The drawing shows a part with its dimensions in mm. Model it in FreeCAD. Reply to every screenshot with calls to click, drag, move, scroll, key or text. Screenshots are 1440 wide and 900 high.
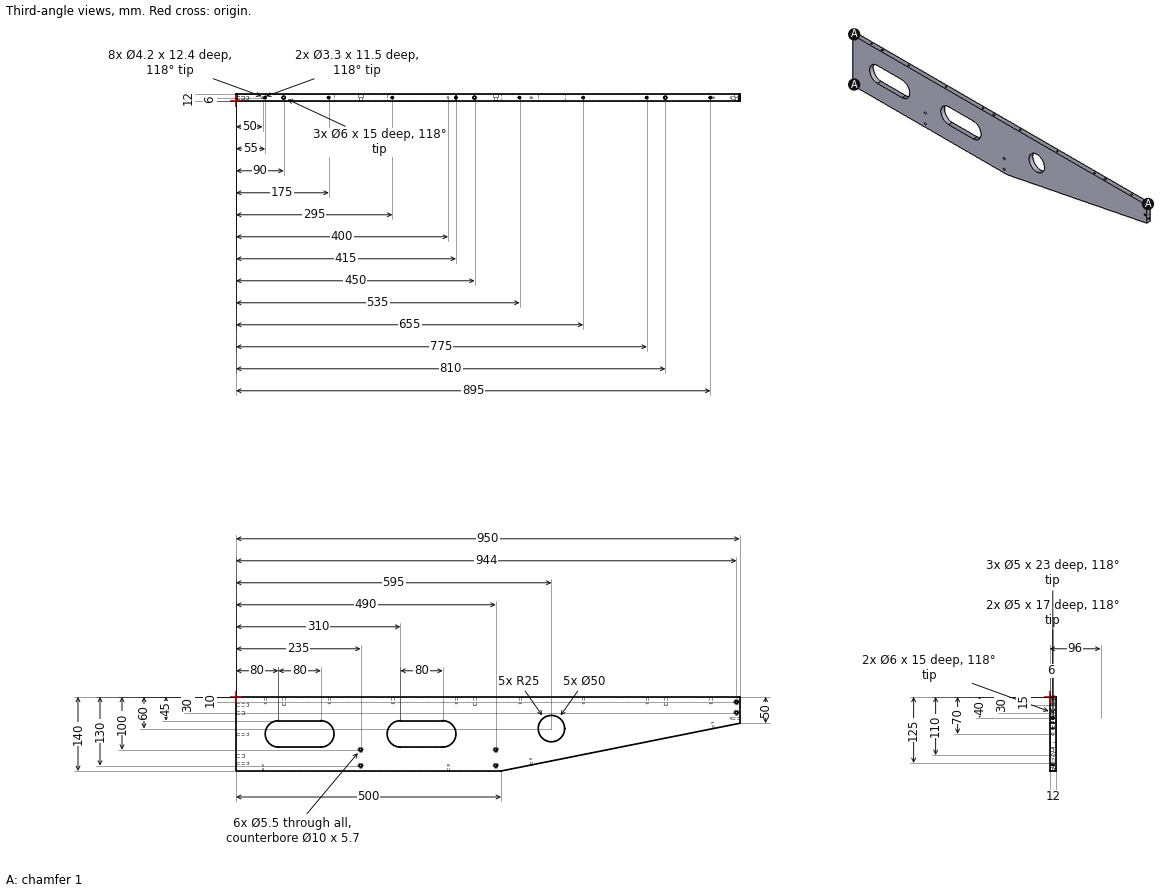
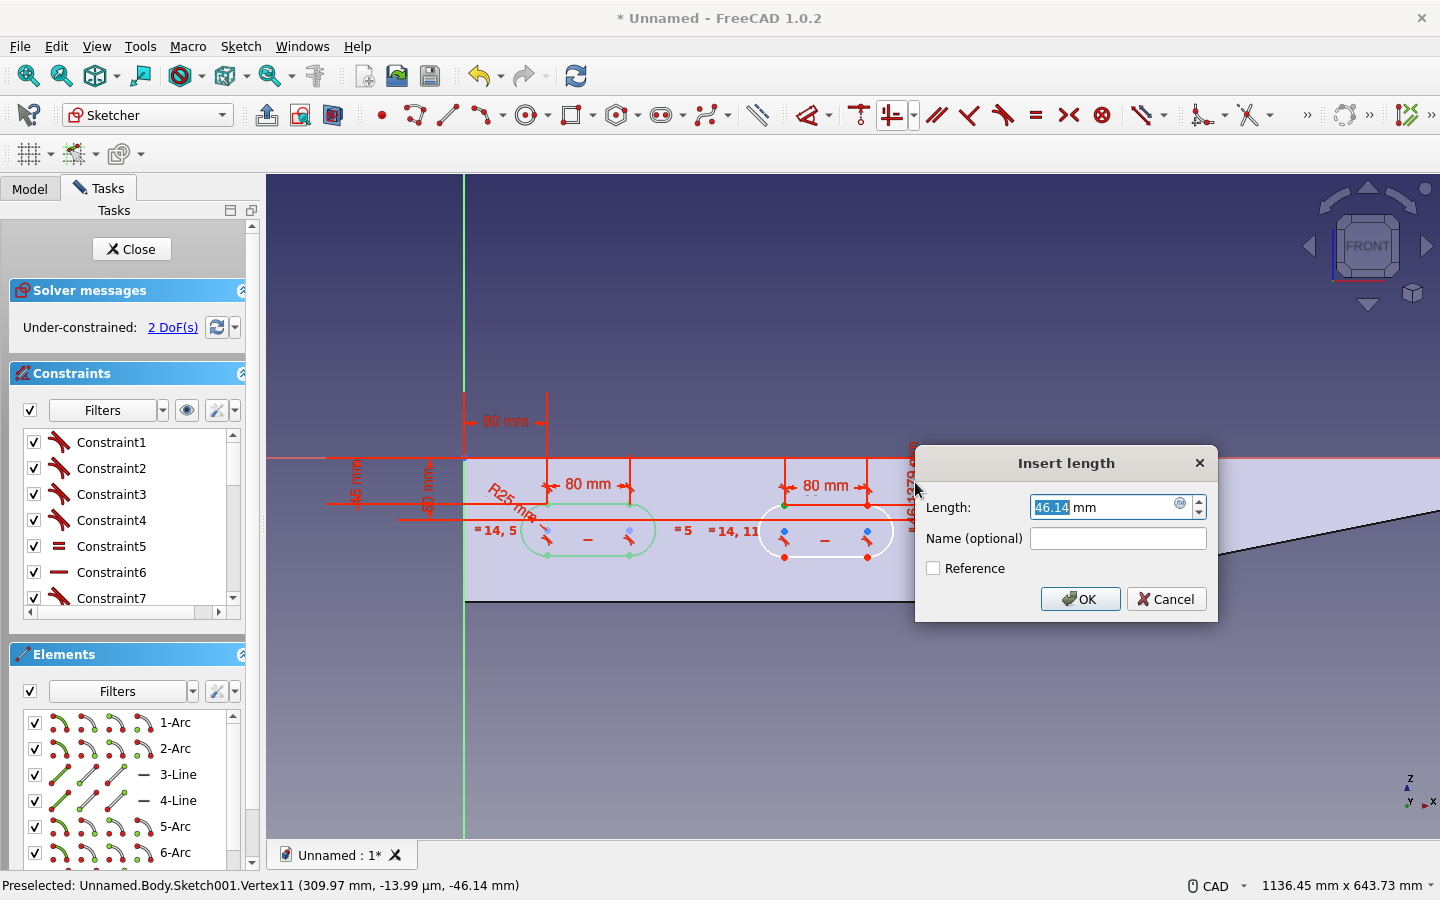
text(45)
key(Return)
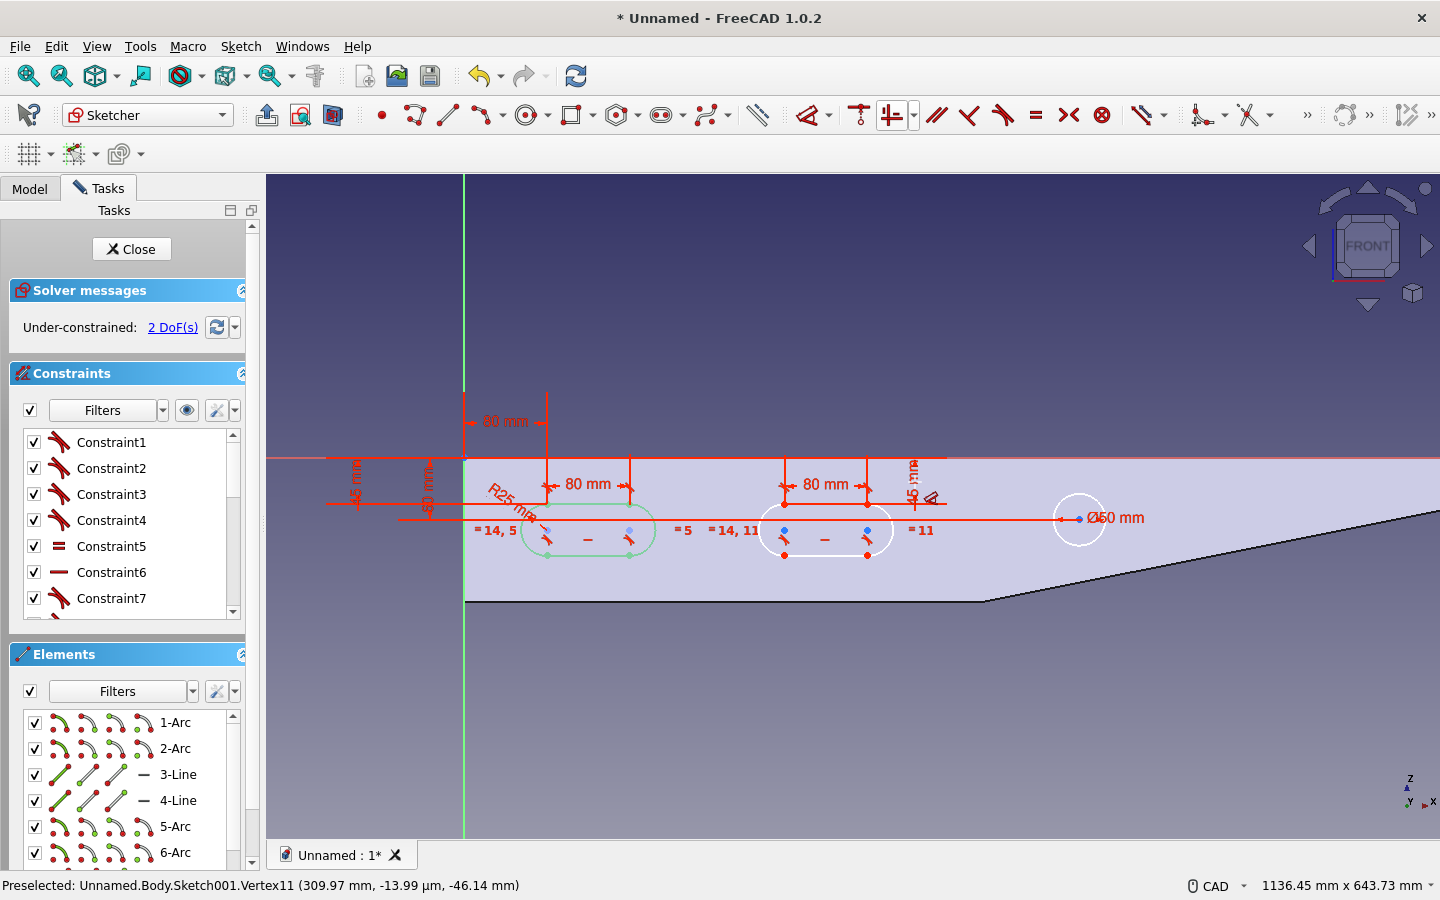
click(1079, 520)
click(772, 424)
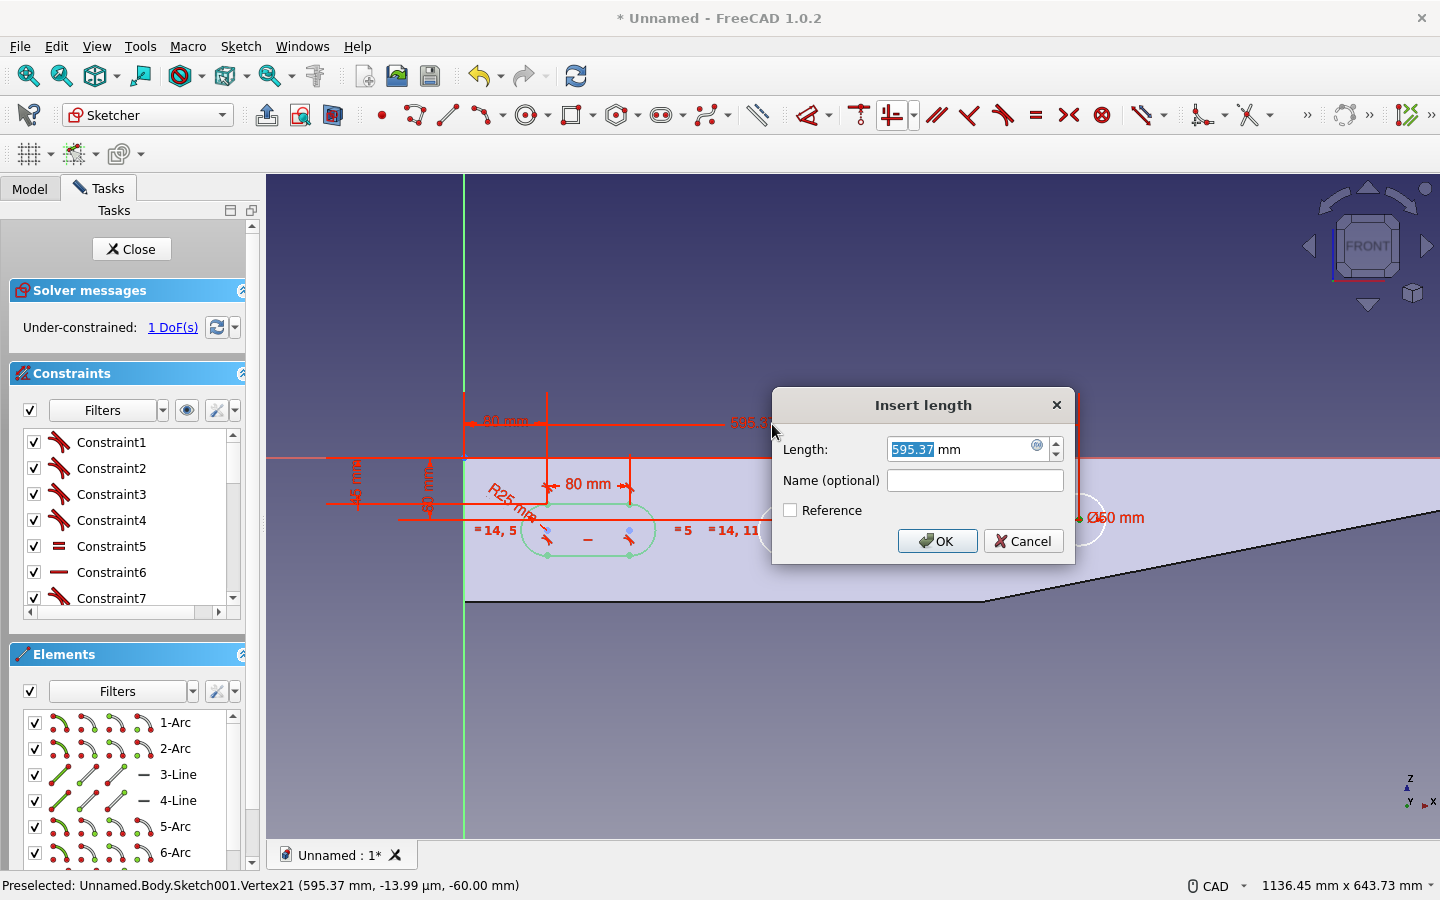
text(595)
key(Return)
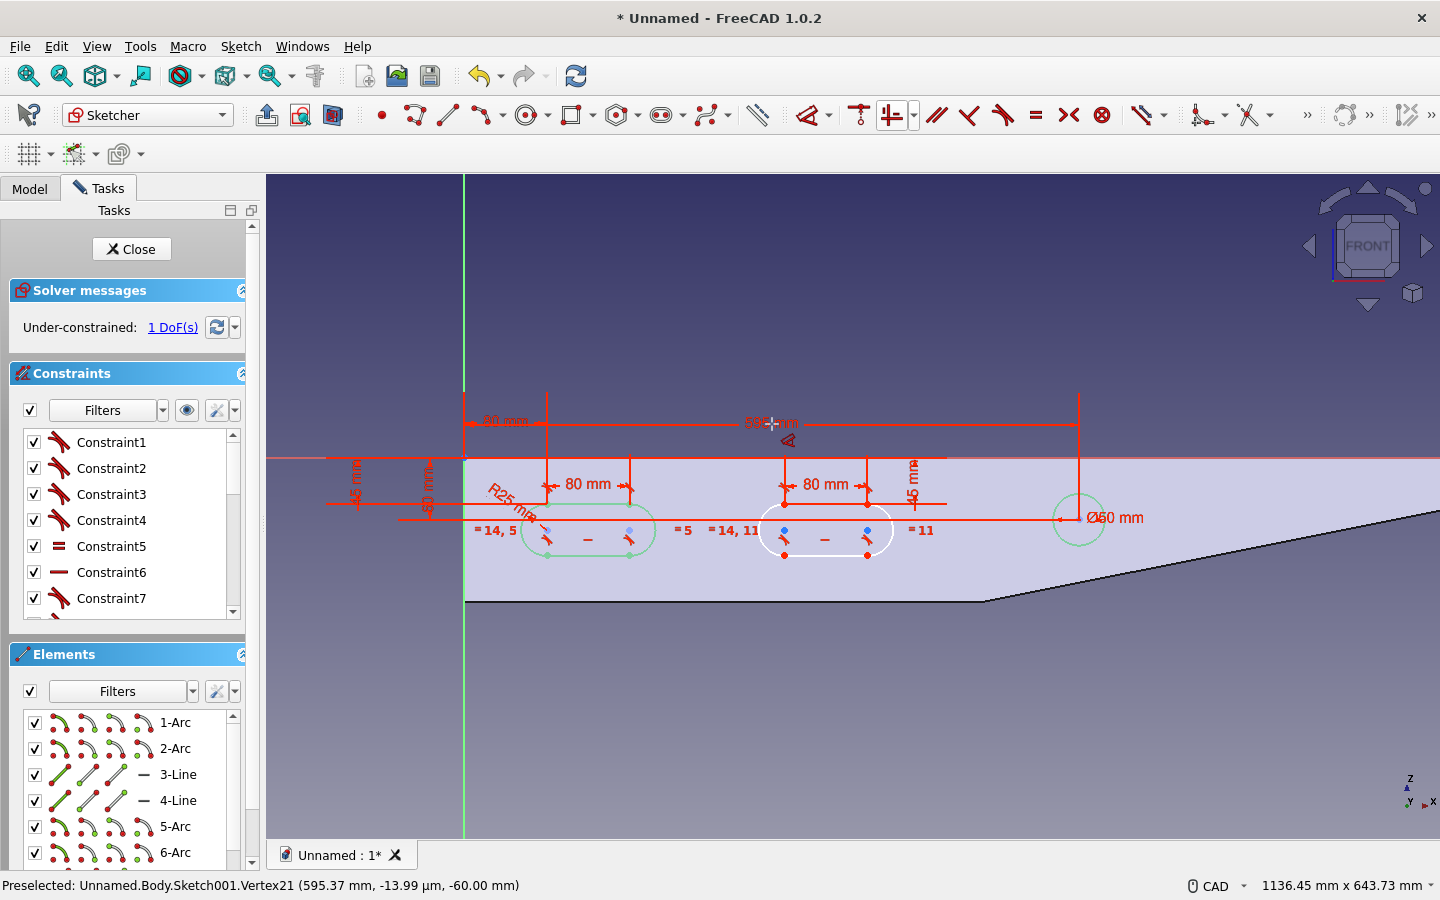
click(785, 504)
click(625, 424)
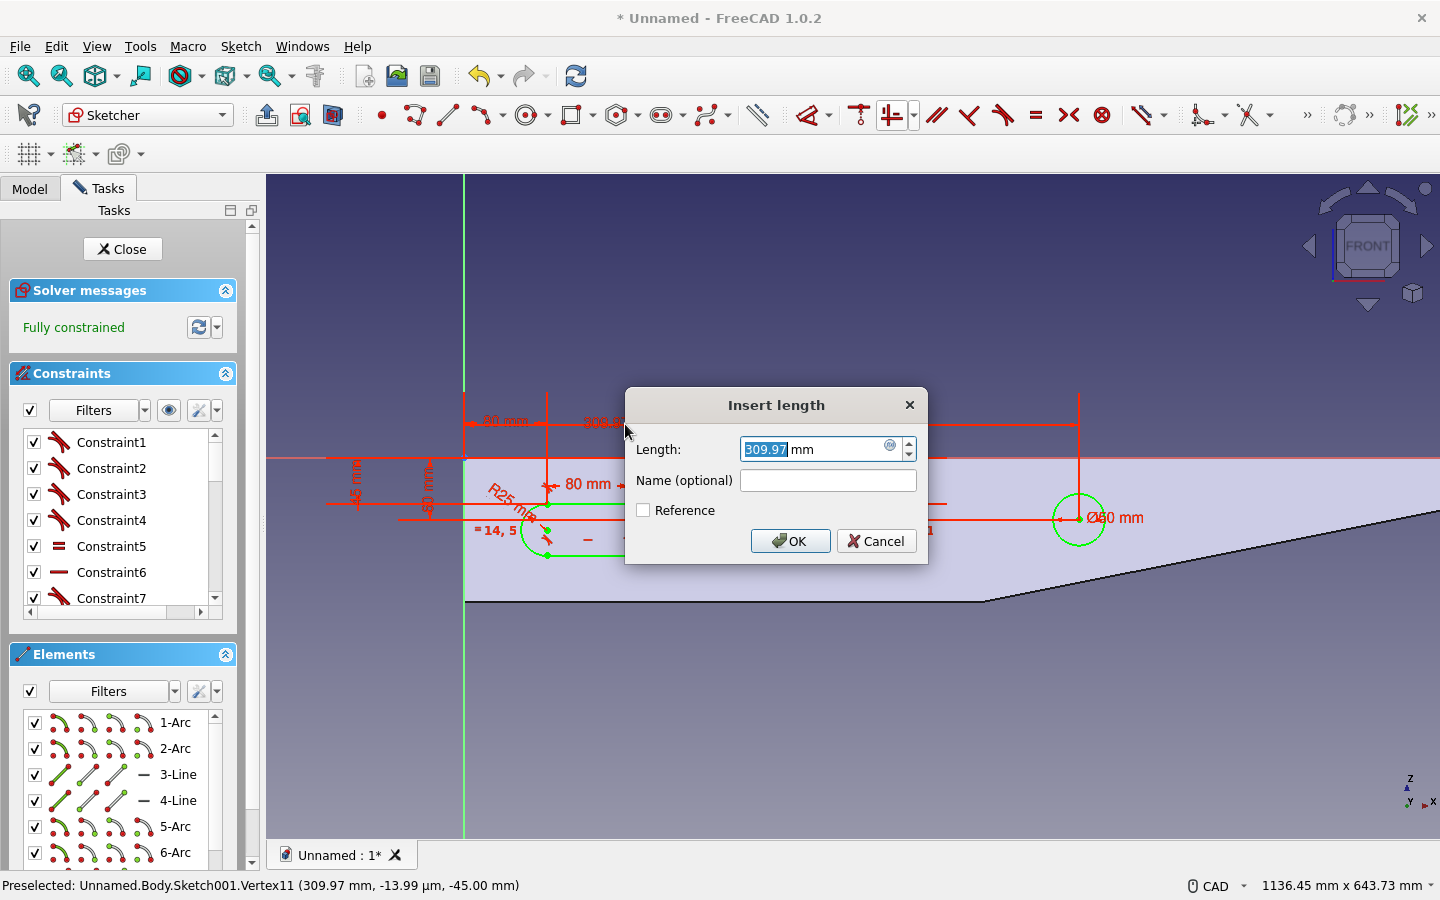
text(310)
key(Return)
key(Escape)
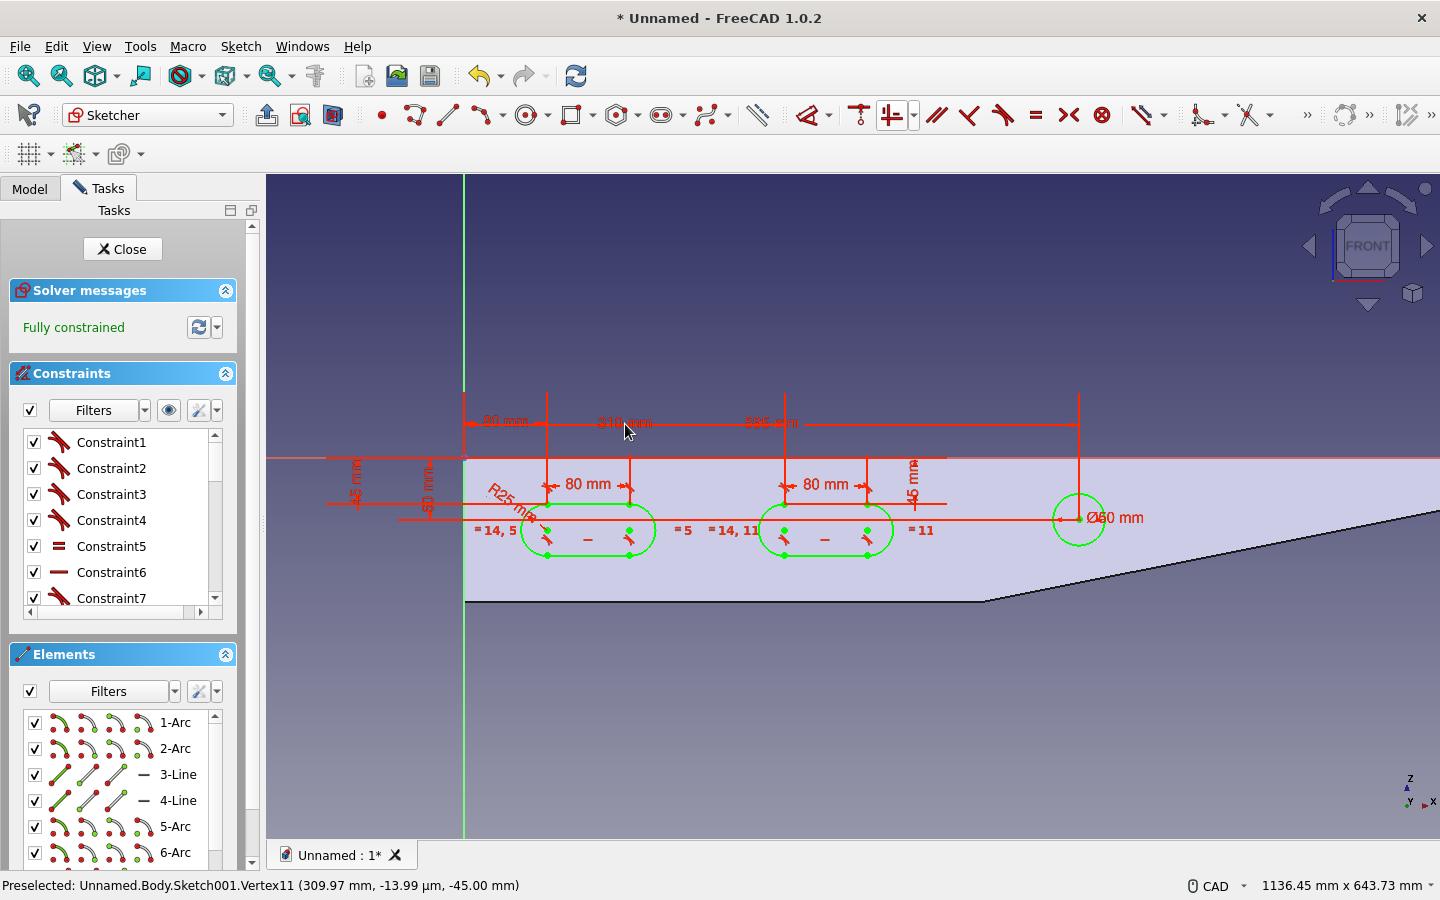
click(123, 249)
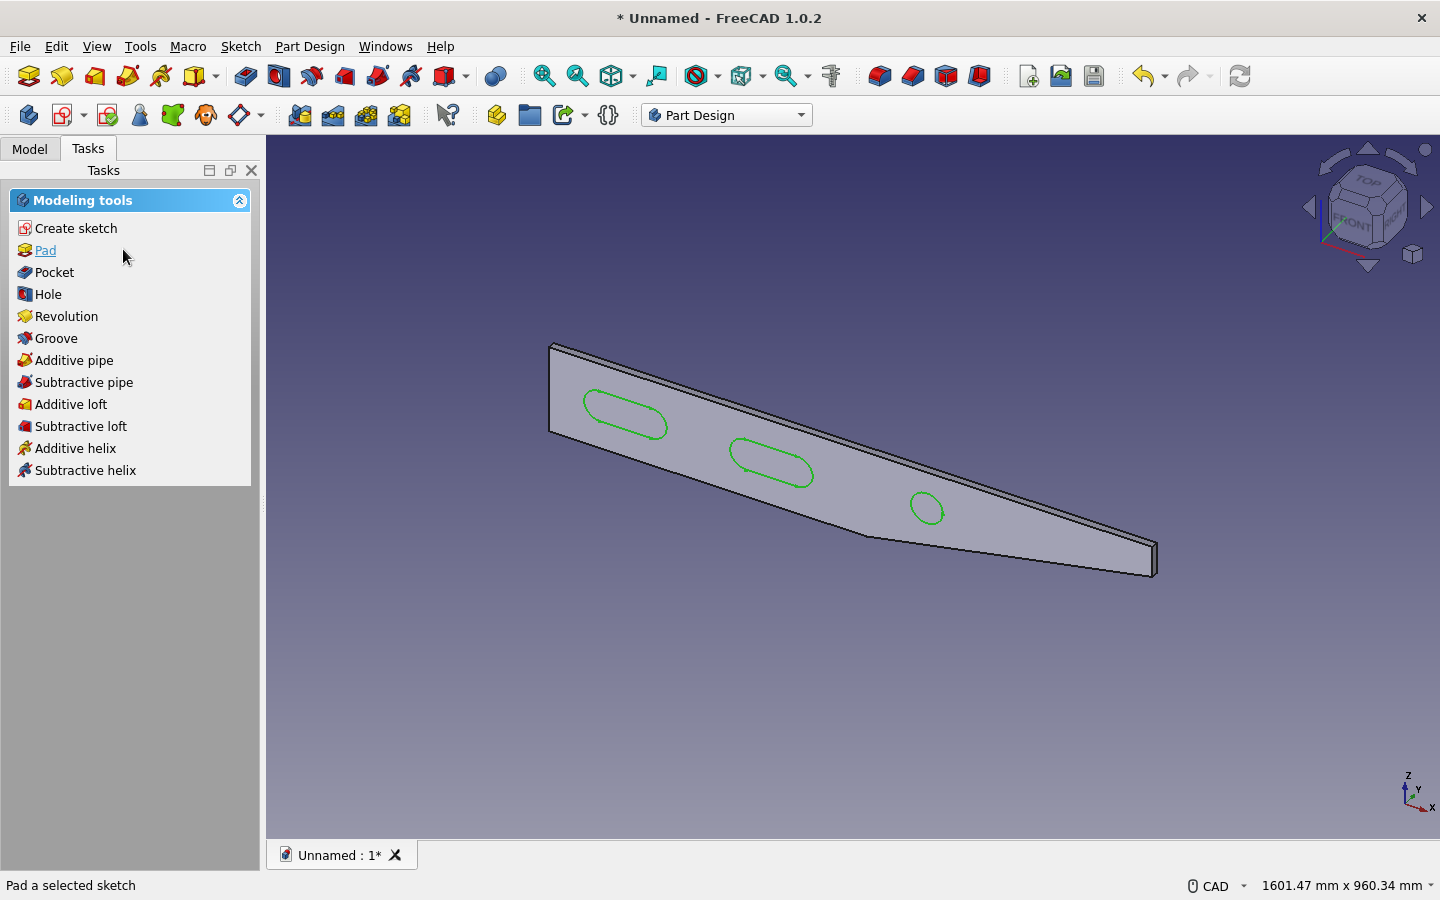
click(246, 76)